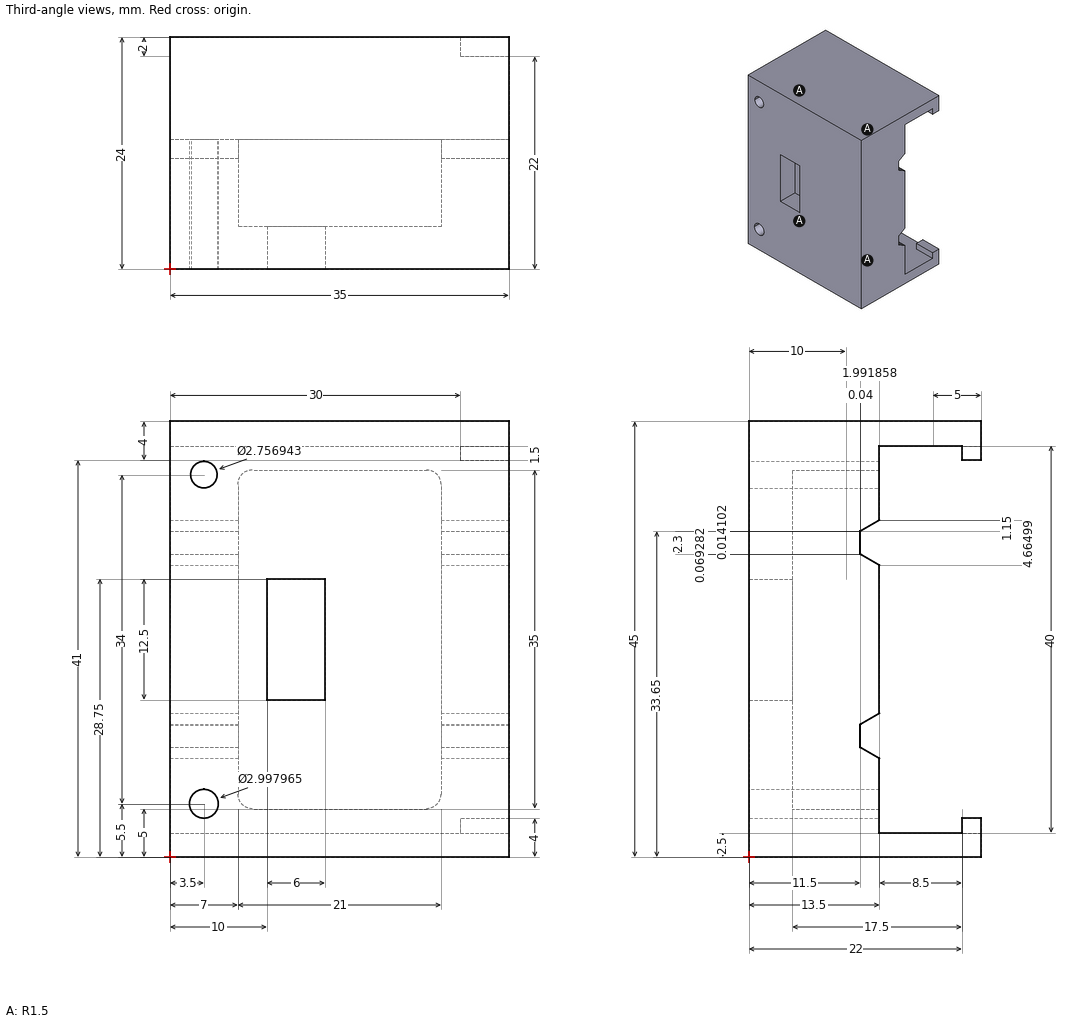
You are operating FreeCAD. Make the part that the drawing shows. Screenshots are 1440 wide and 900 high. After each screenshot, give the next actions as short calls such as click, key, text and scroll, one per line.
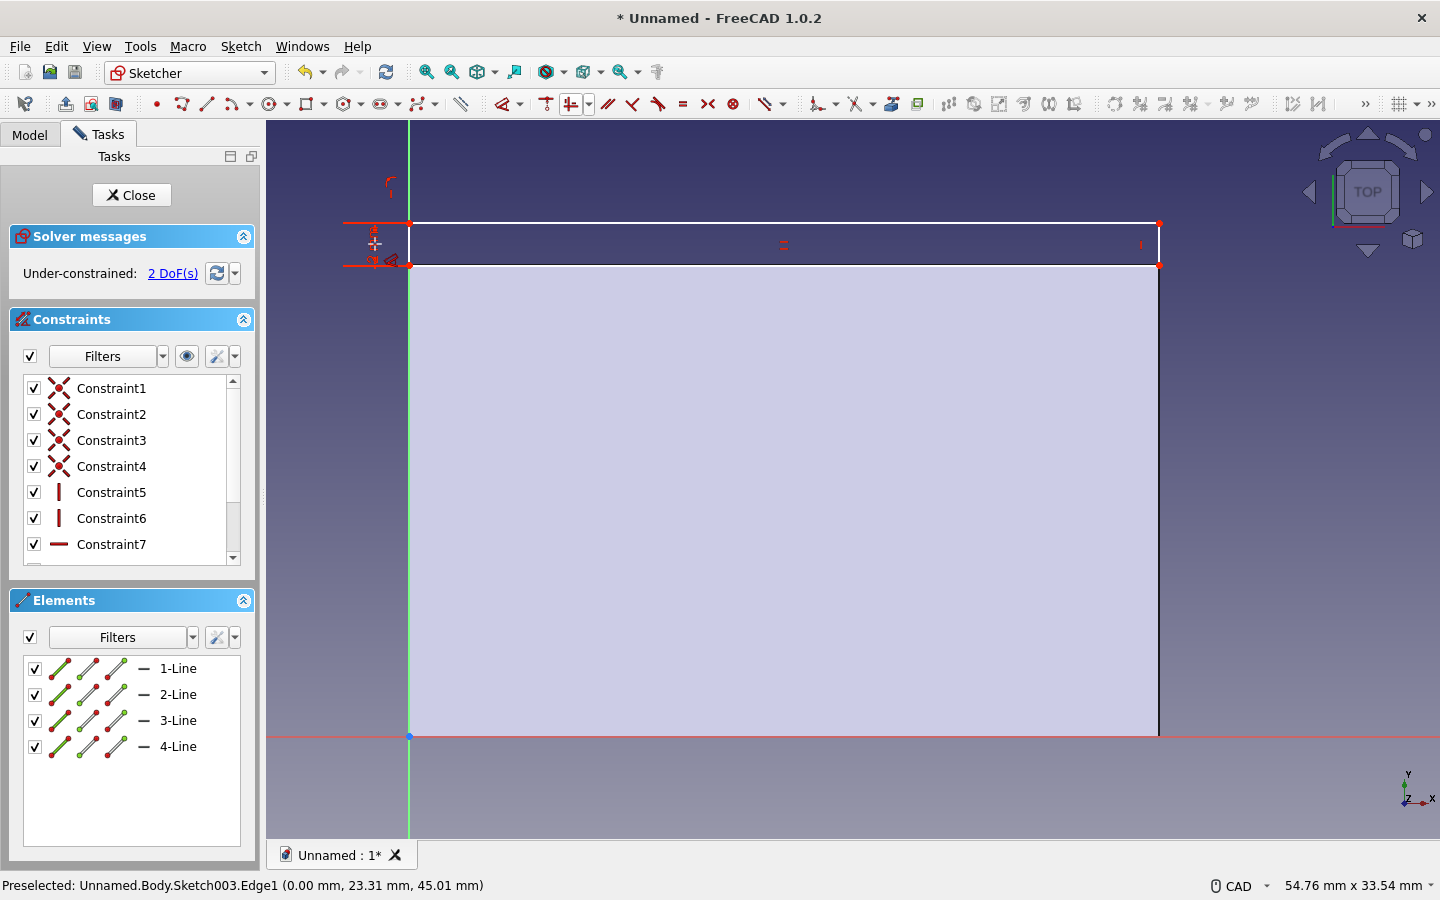
click(634, 266)
click(784, 300)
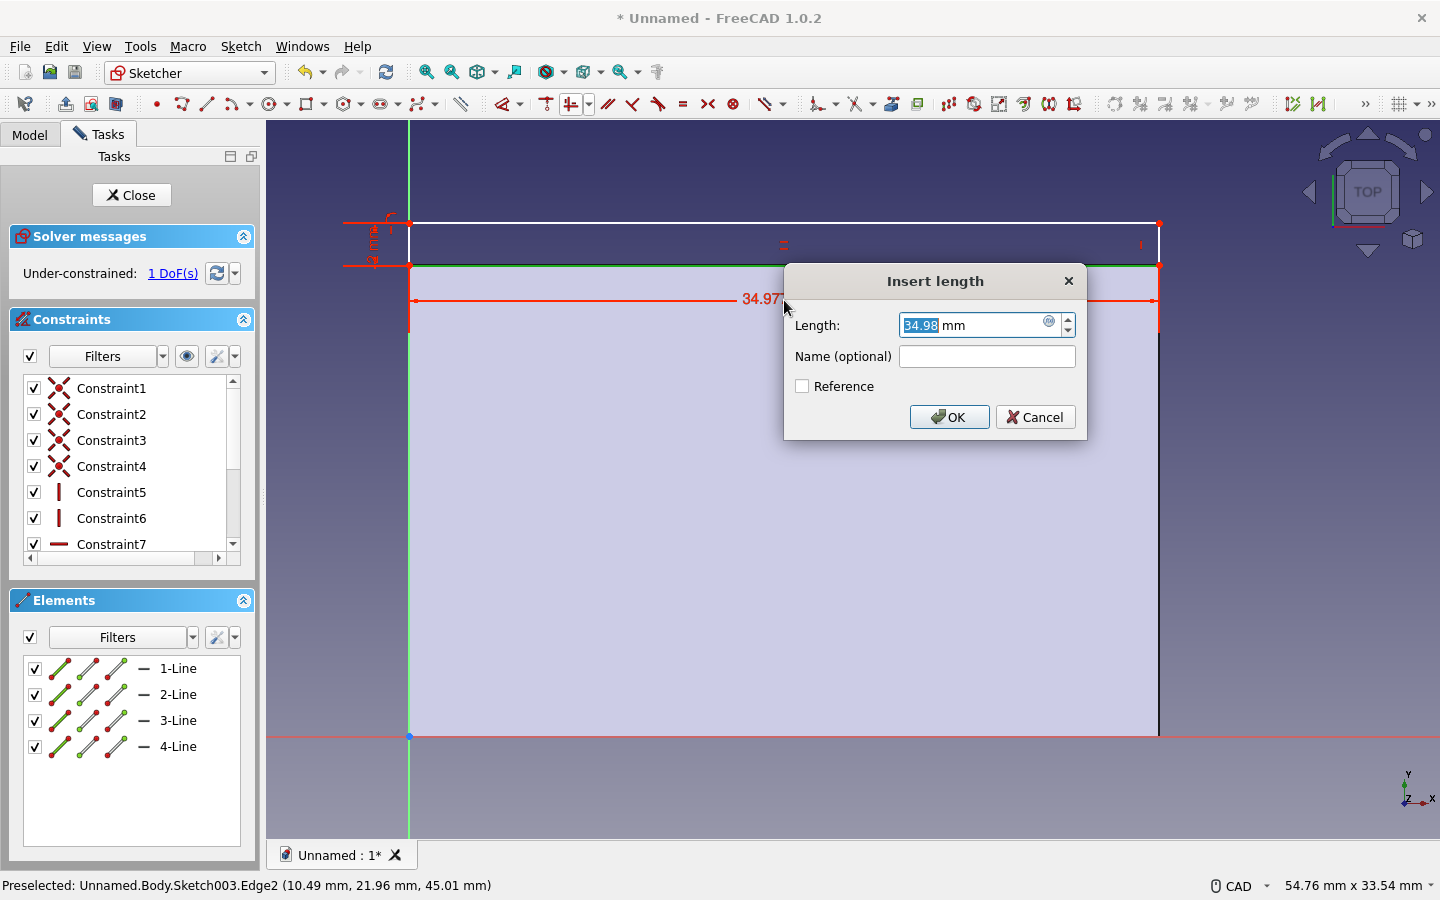
text(35)
key(Return)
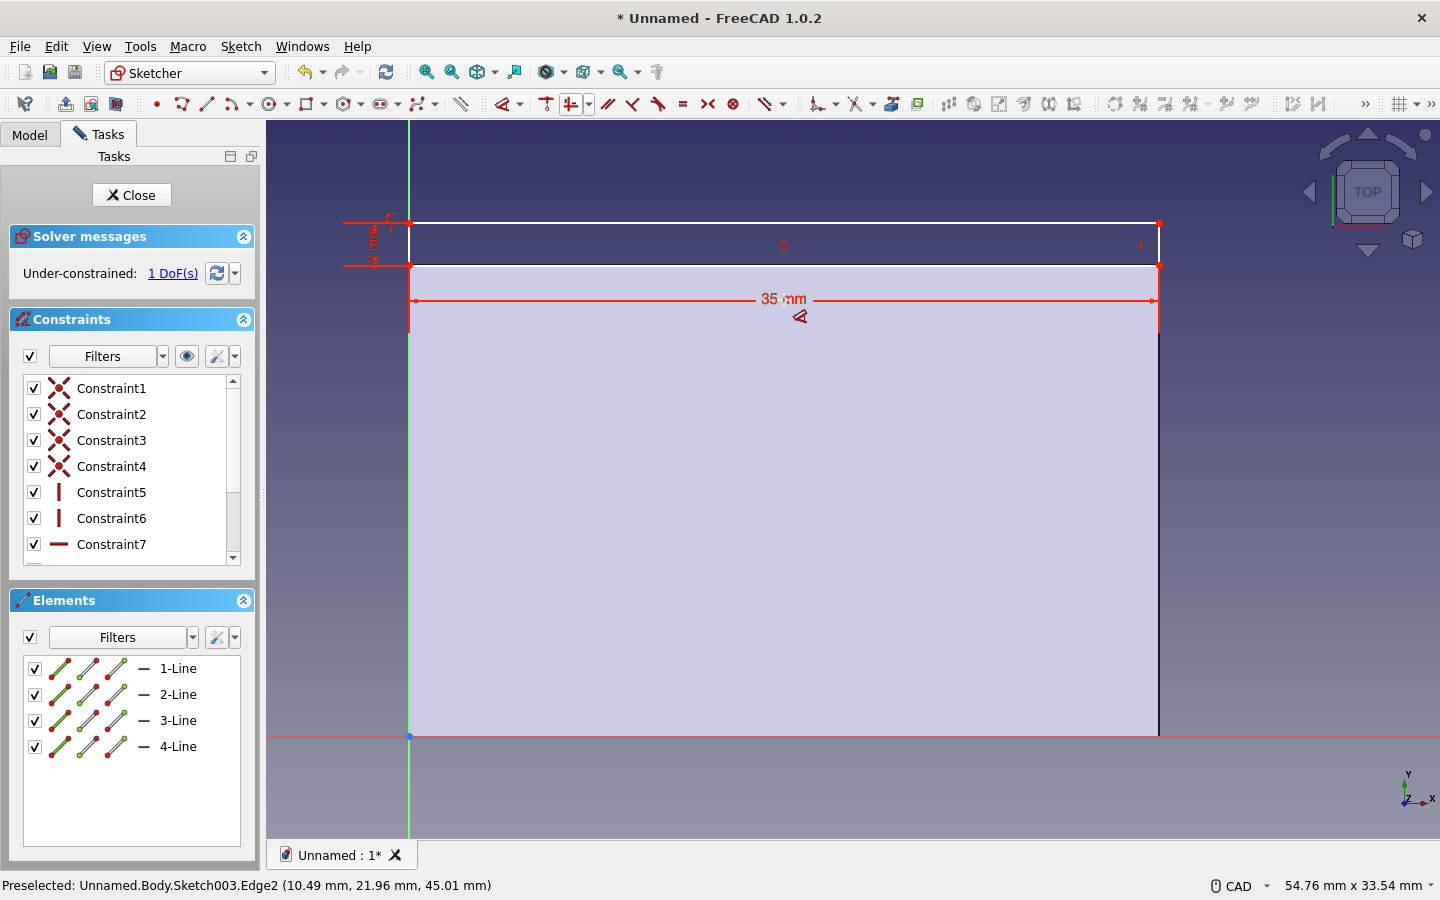
click(409, 223)
click(375, 480)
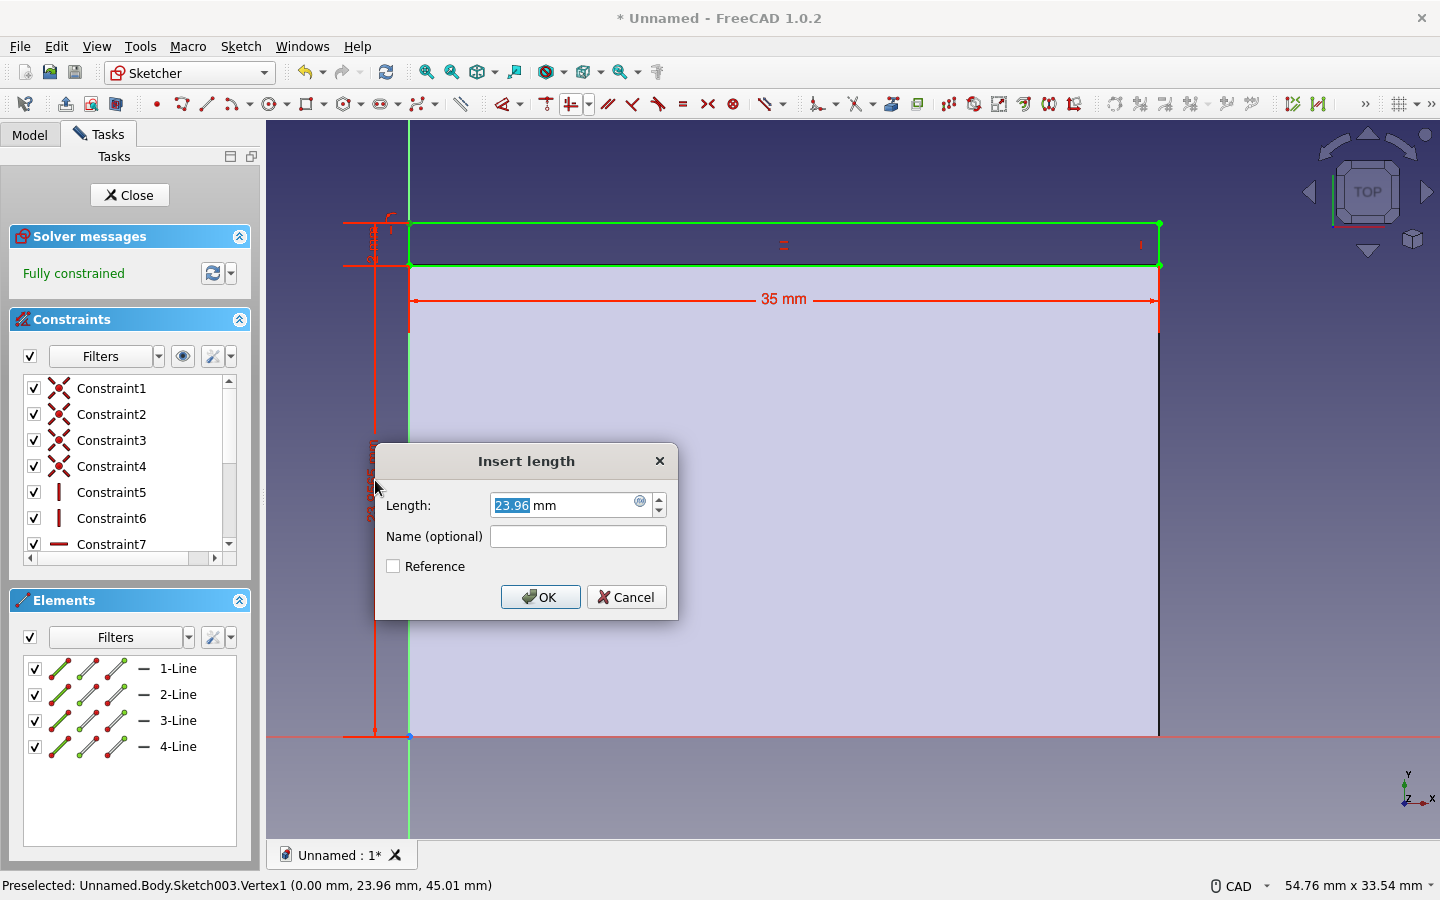
text(24)
key(Return)
key(Escape)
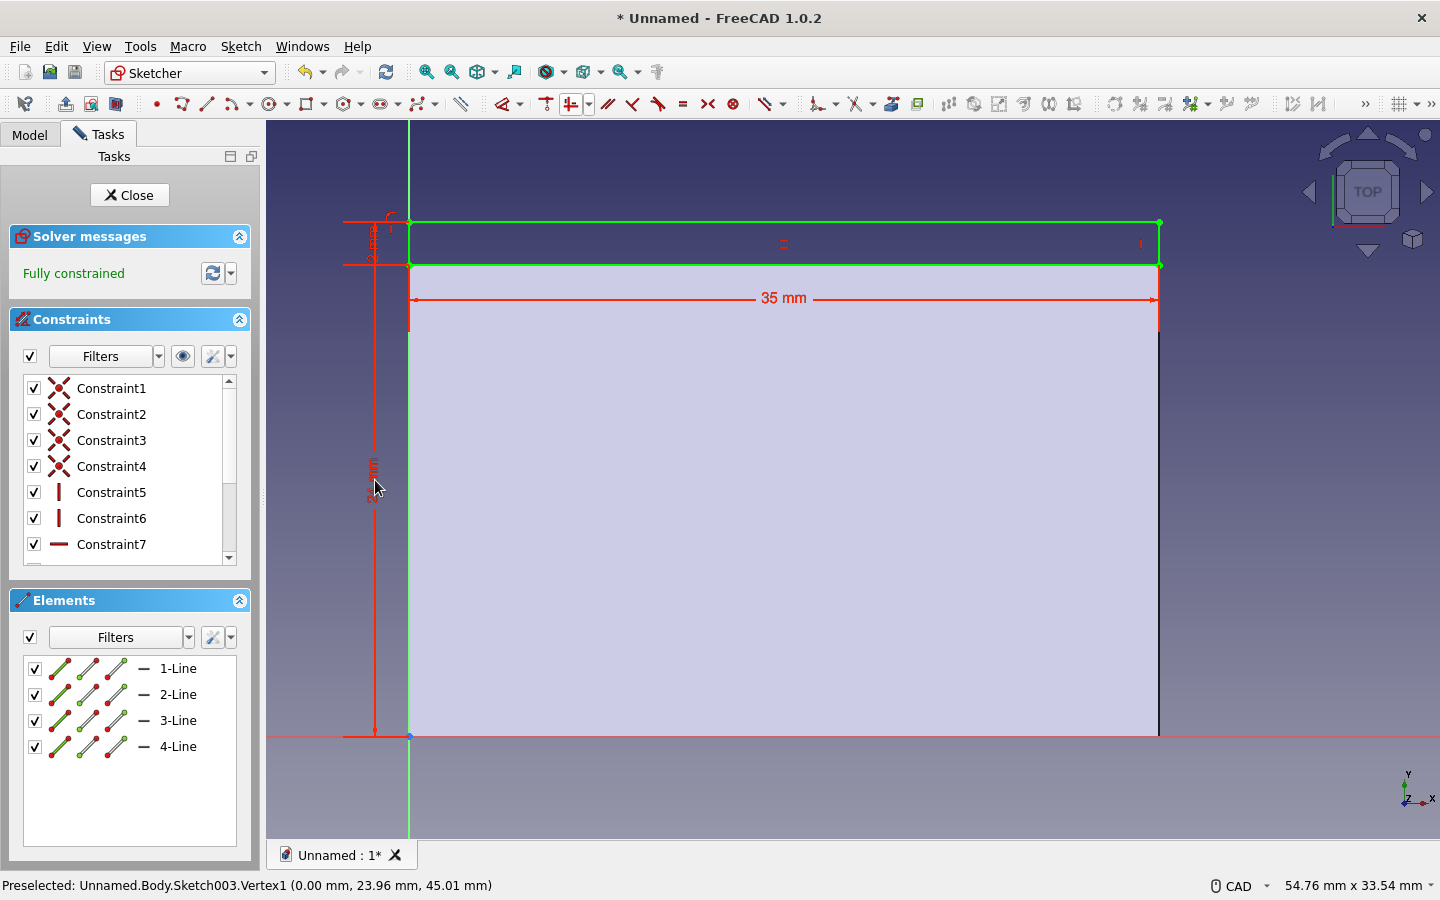
click(130, 195)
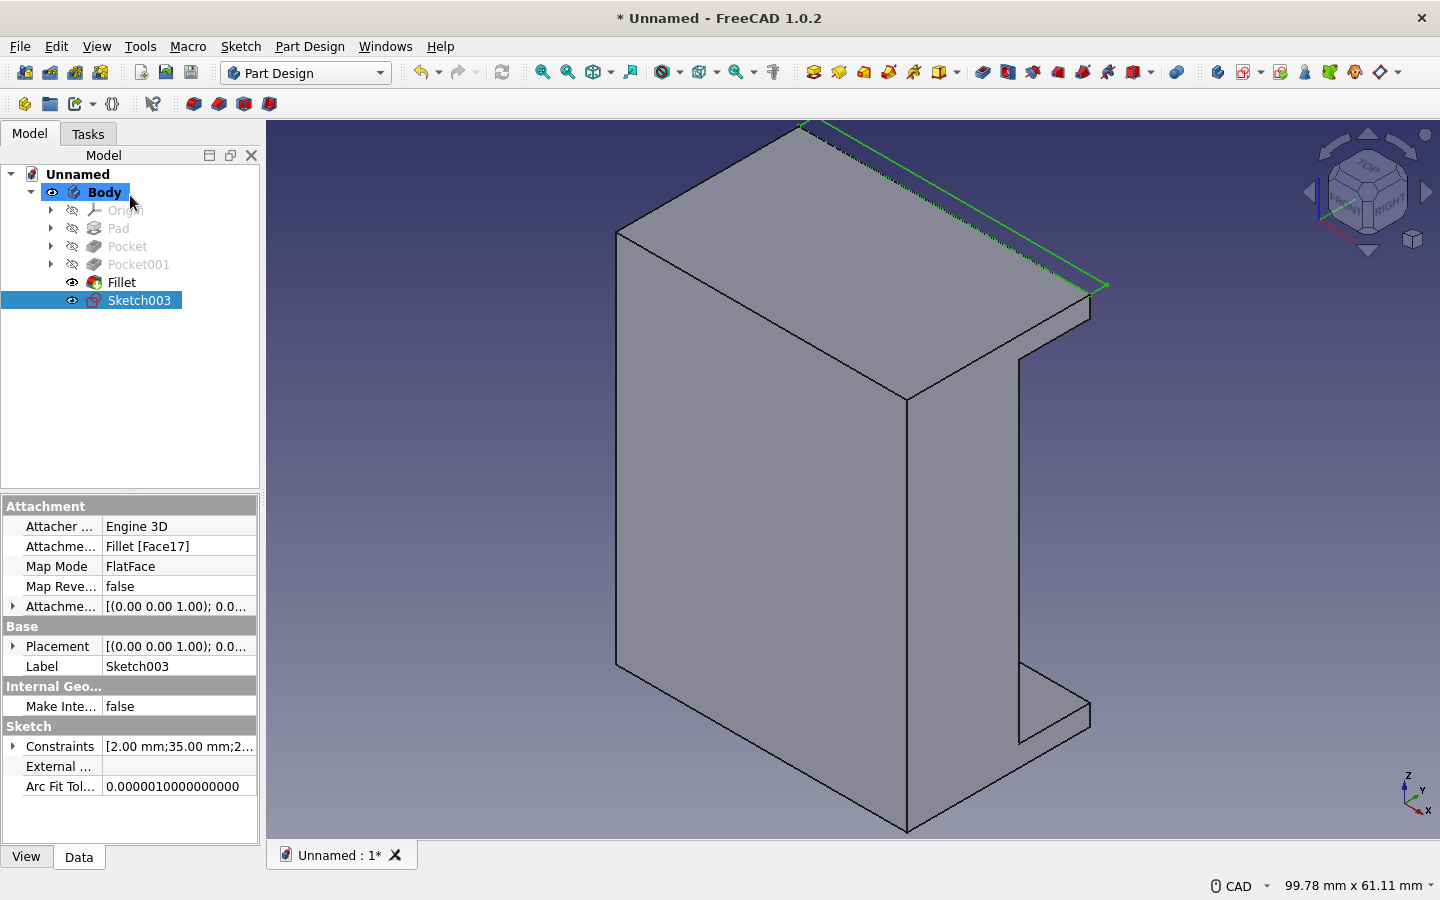
click(814, 72)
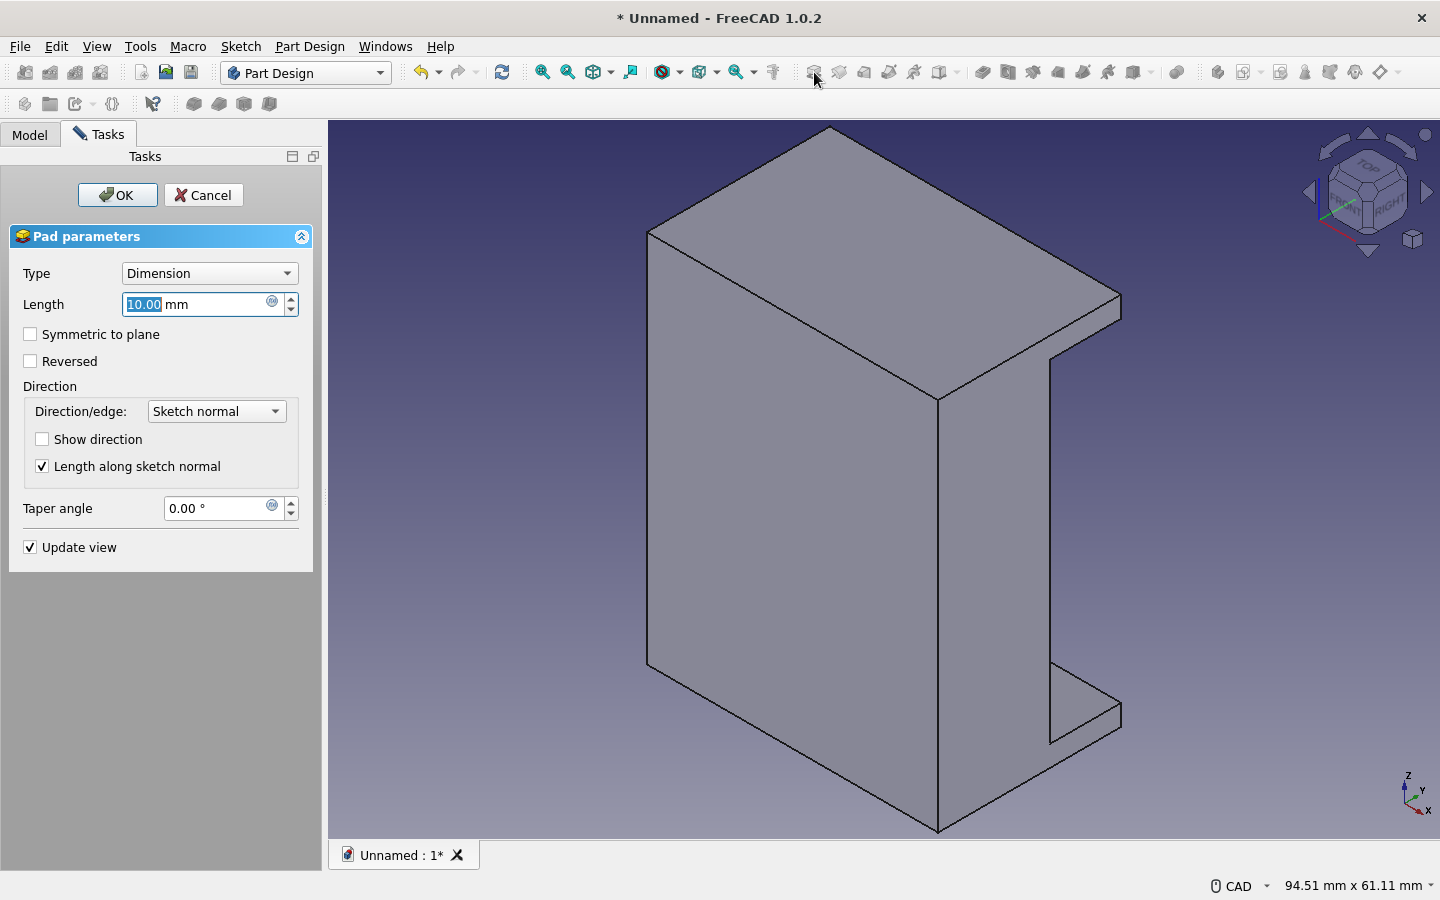
text(4)
key(Tab)